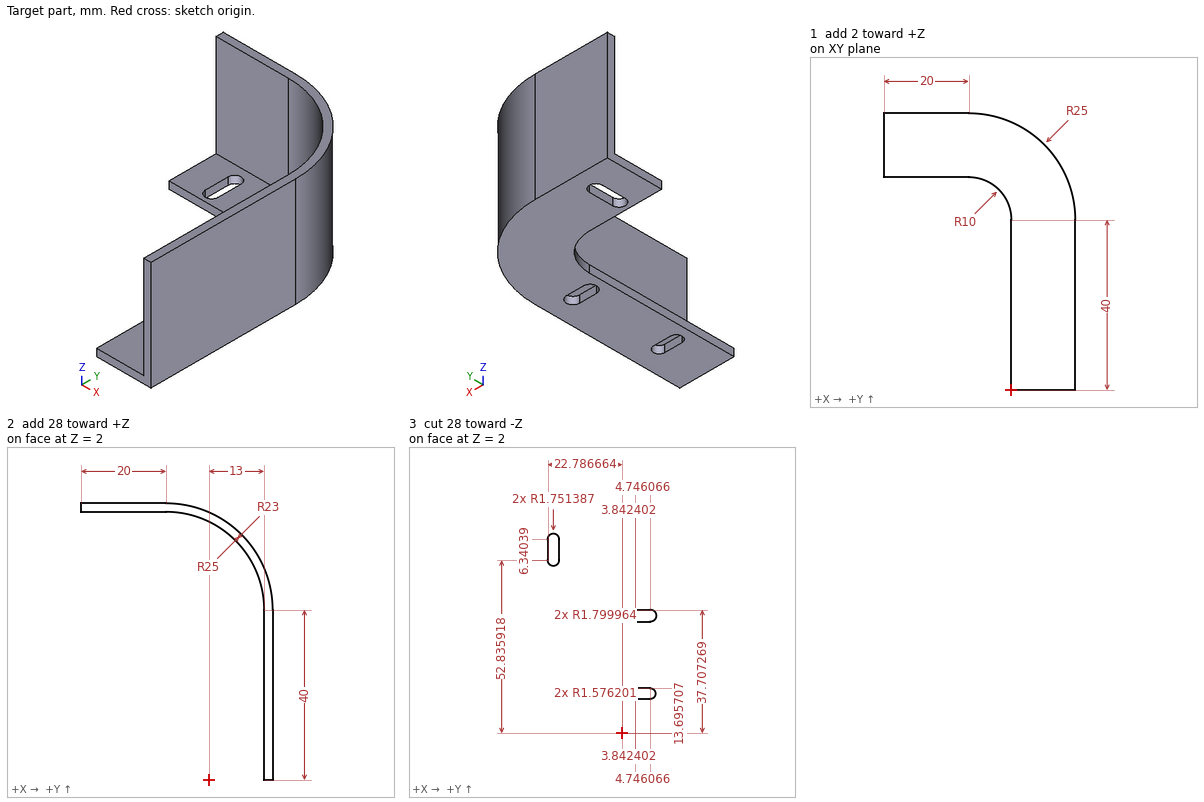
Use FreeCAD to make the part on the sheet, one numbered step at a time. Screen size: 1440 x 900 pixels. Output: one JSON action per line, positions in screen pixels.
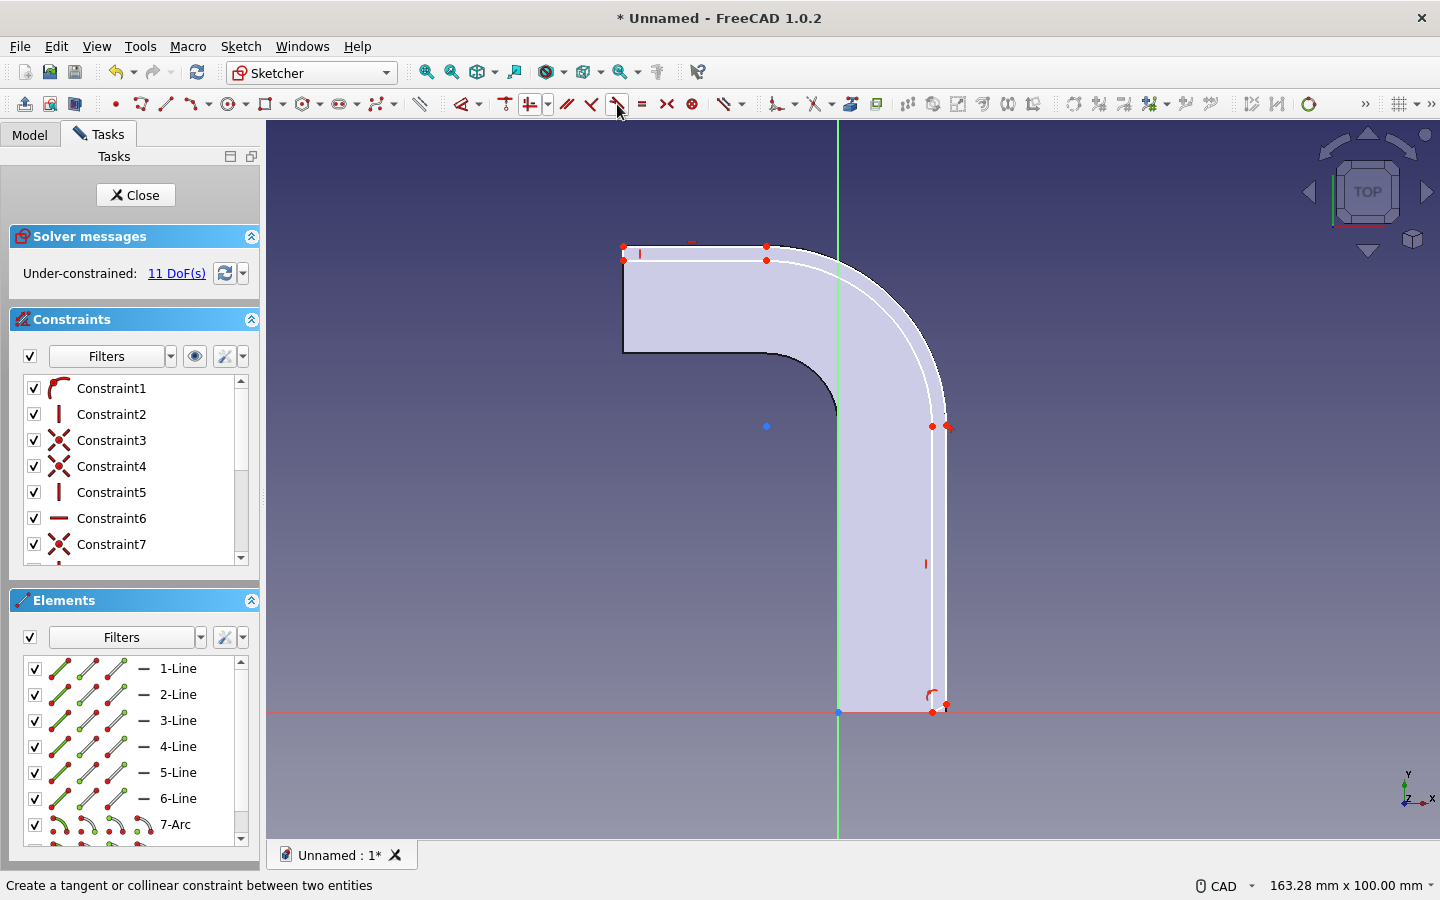
{"action": "left_click", "coordinate": [946, 621]}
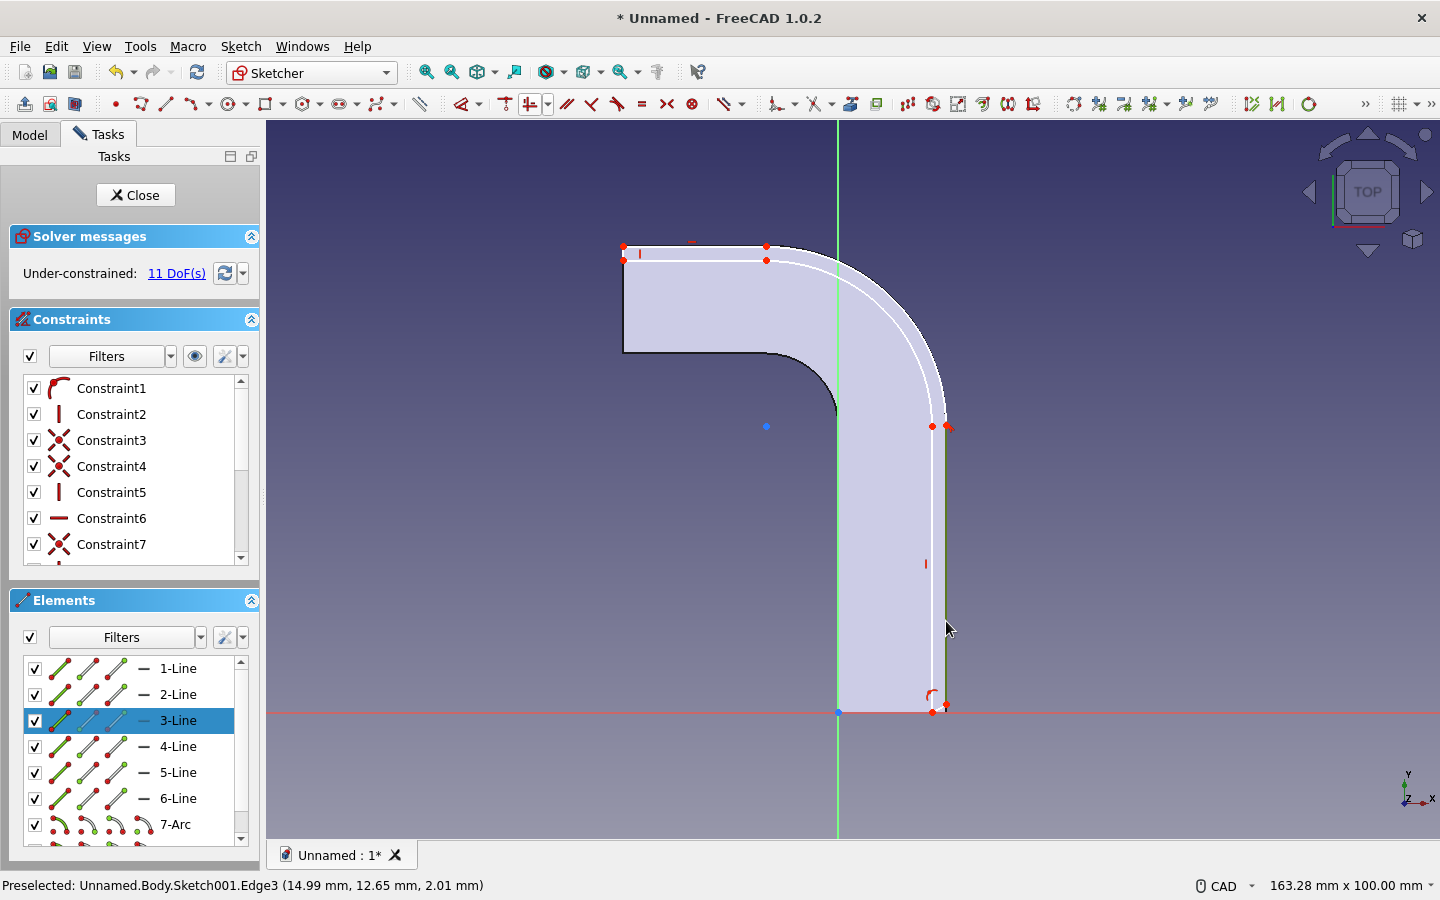
{"action": "left_click", "coordinate": [926, 345]}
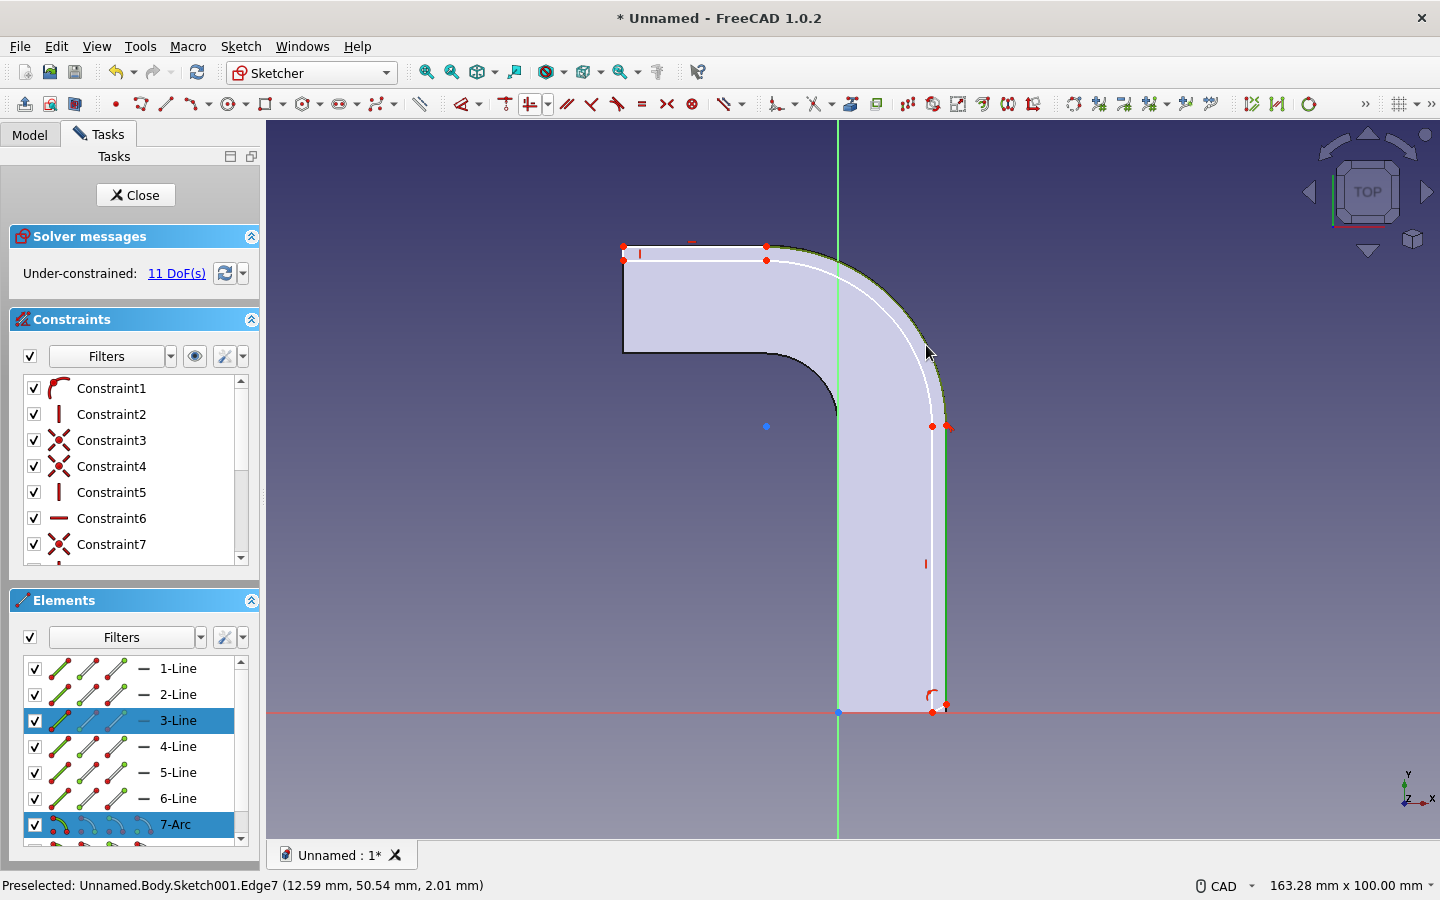
{"action": "left_click", "coordinate": [617, 104]}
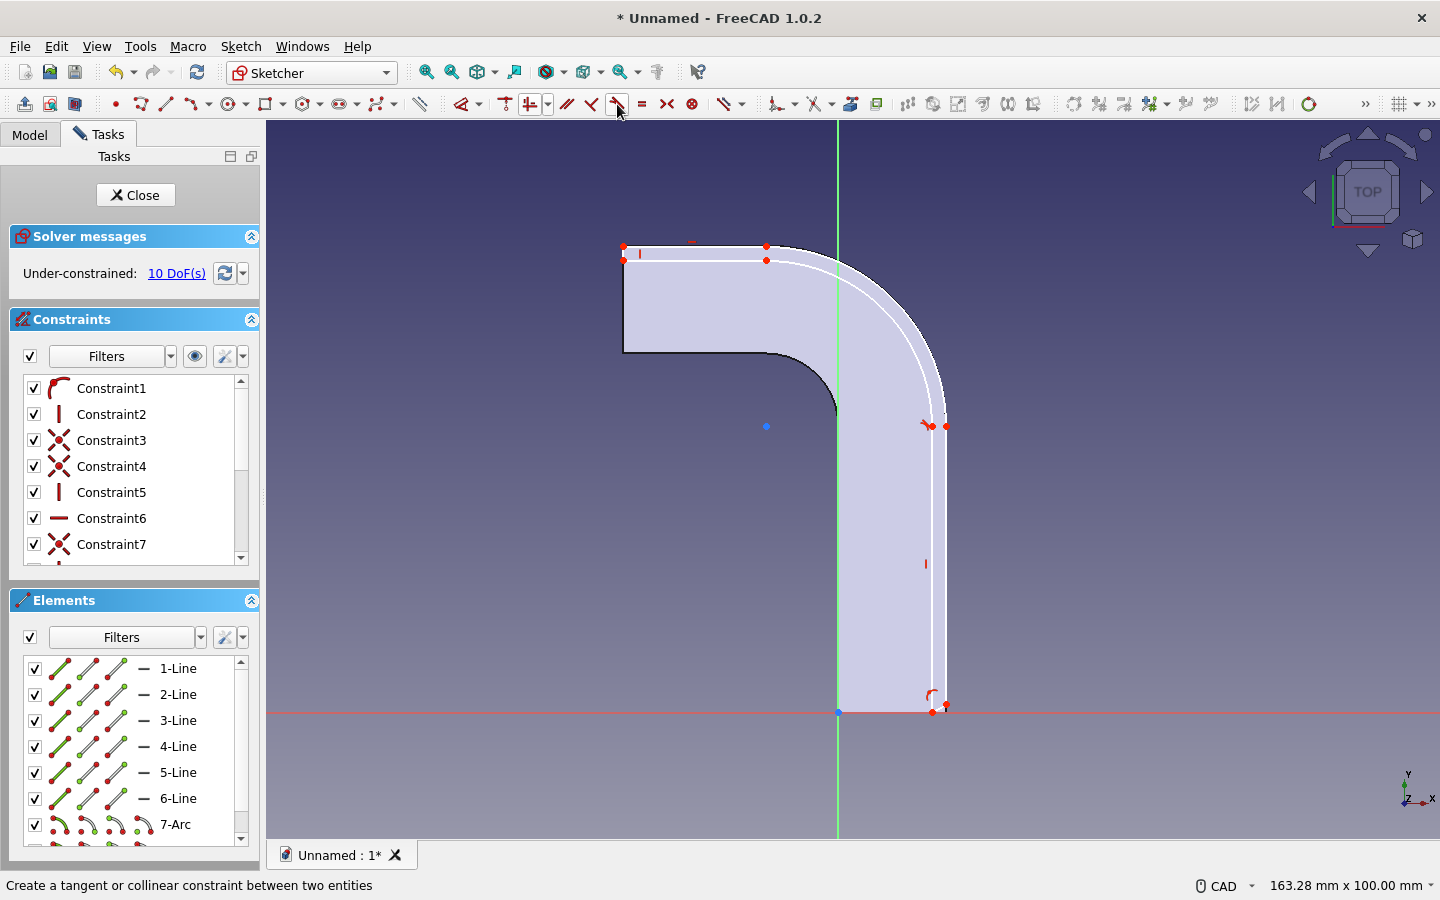
{"action": "left_click", "coordinate": [723, 247]}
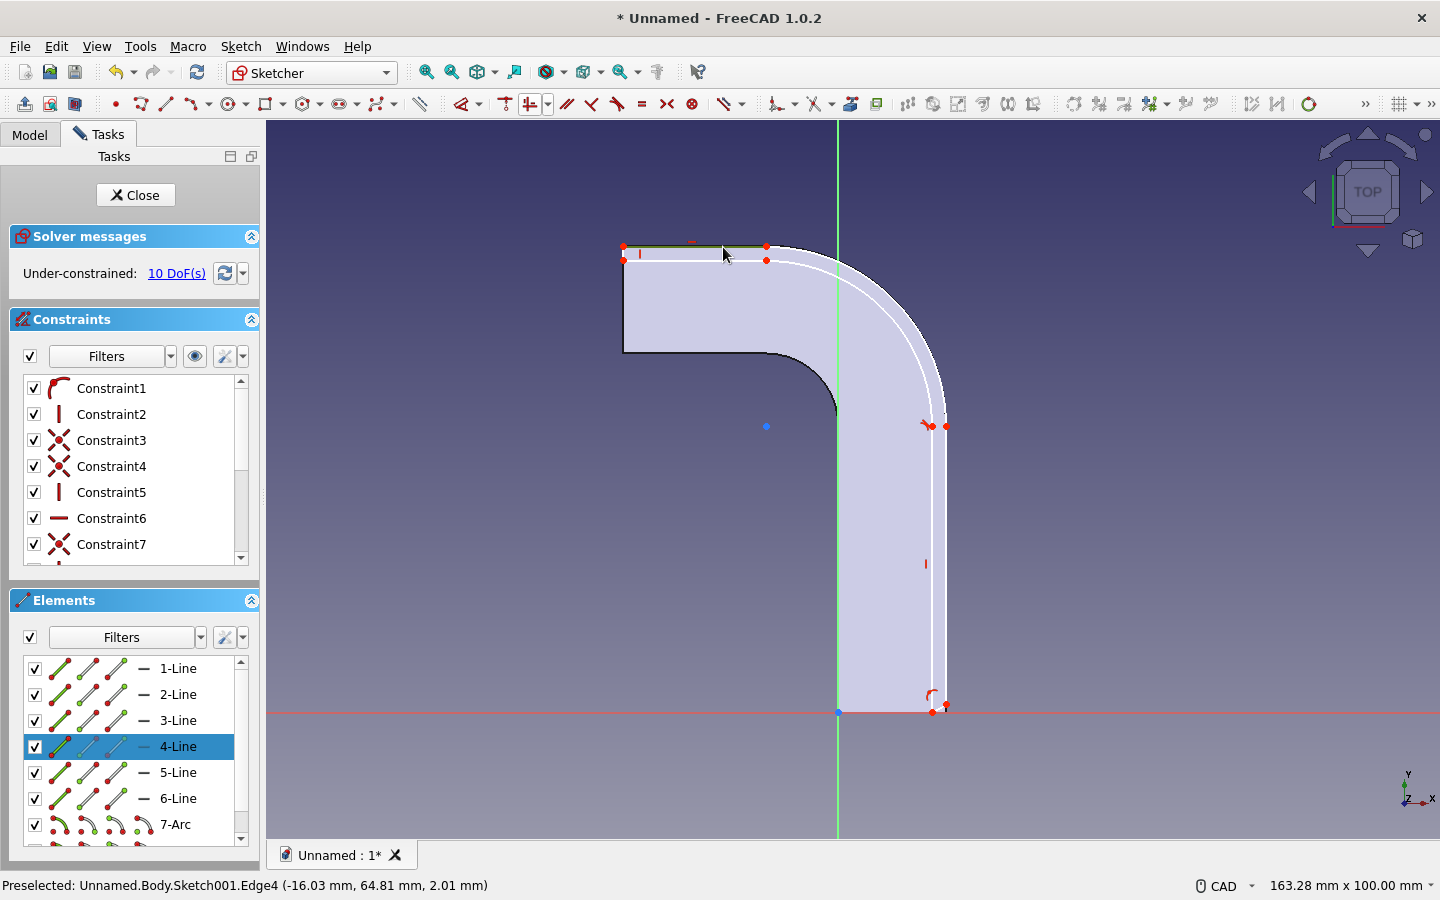
{"action": "left_click", "coordinate": [926, 345]}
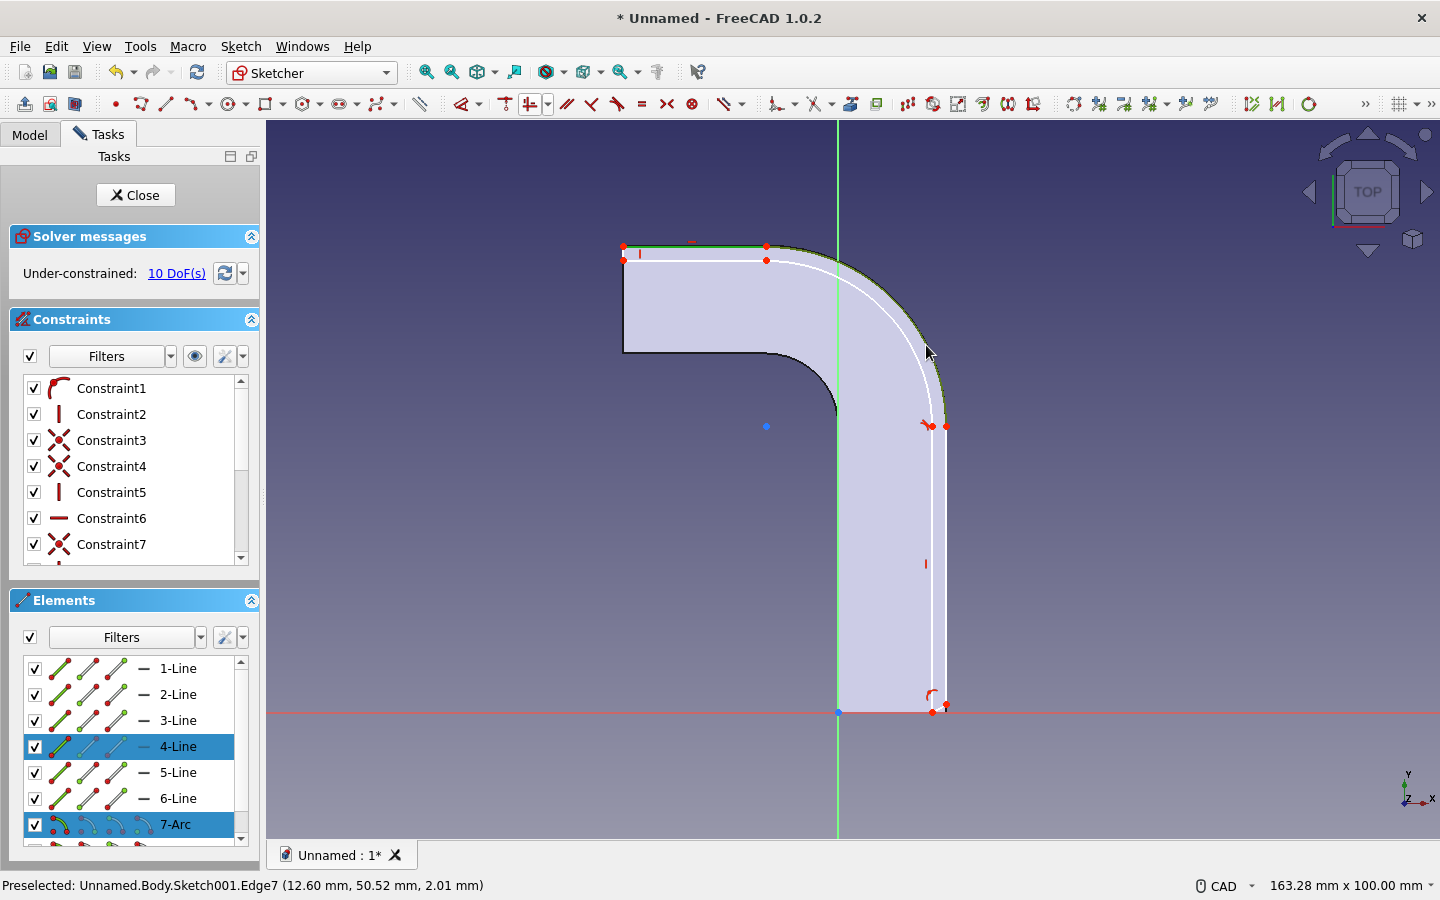
{"action": "left_click", "coordinate": [617, 104]}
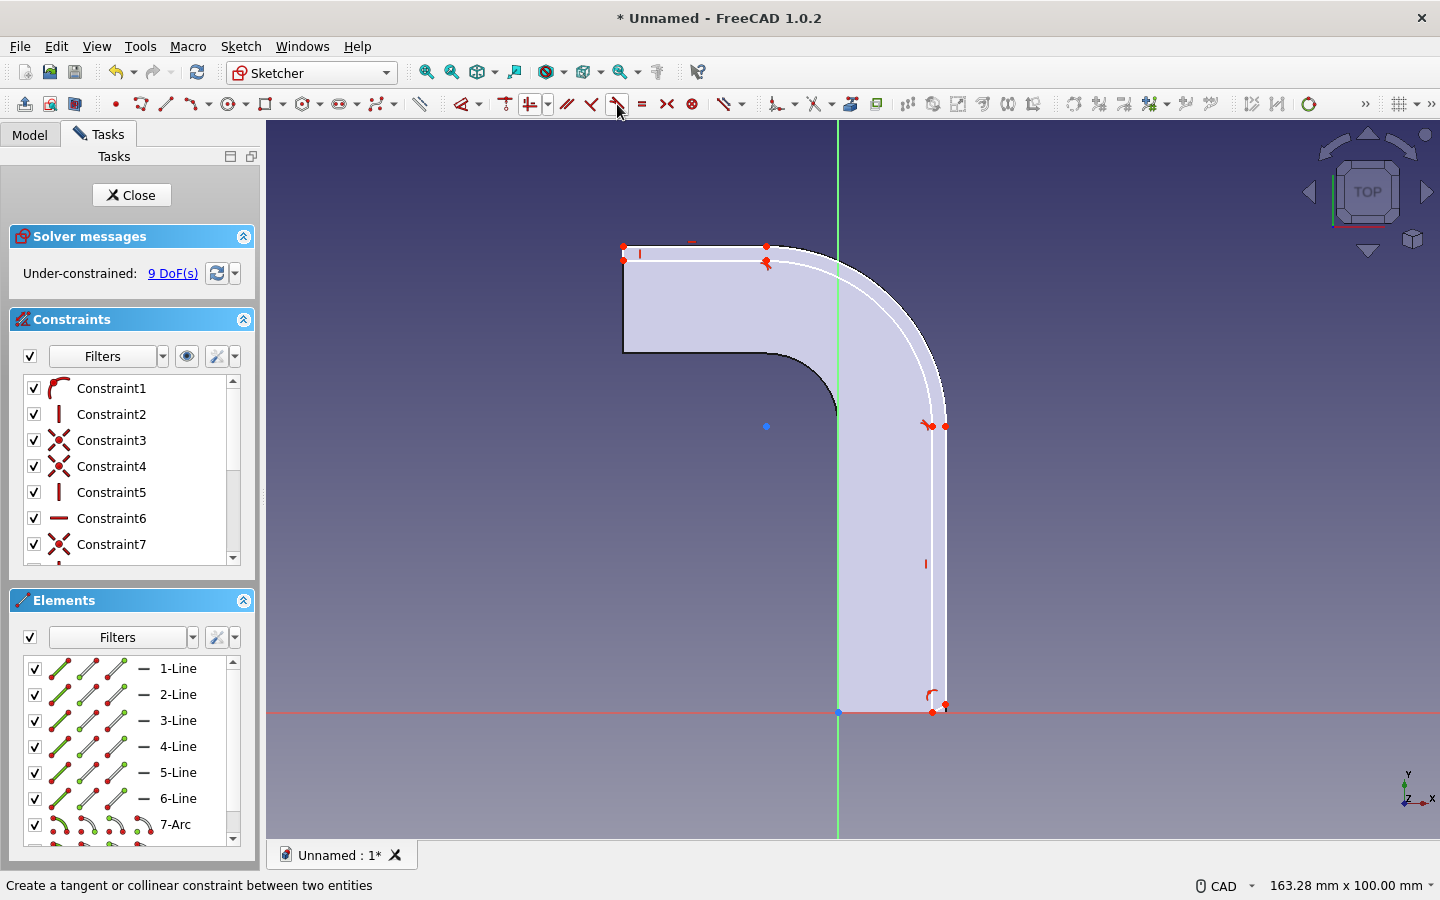
{"action": "left_click", "coordinate": [666, 261]}